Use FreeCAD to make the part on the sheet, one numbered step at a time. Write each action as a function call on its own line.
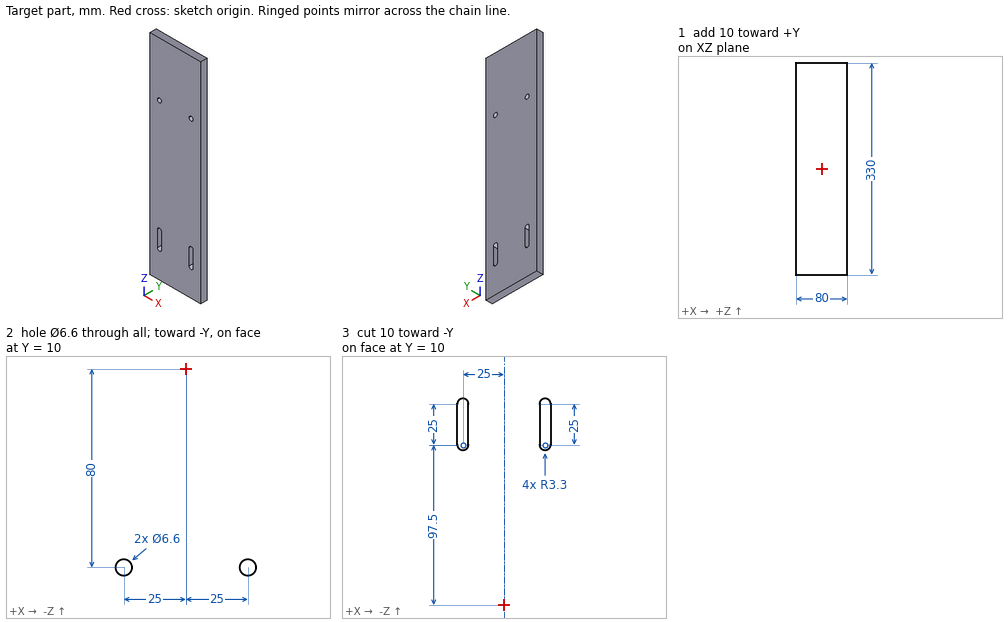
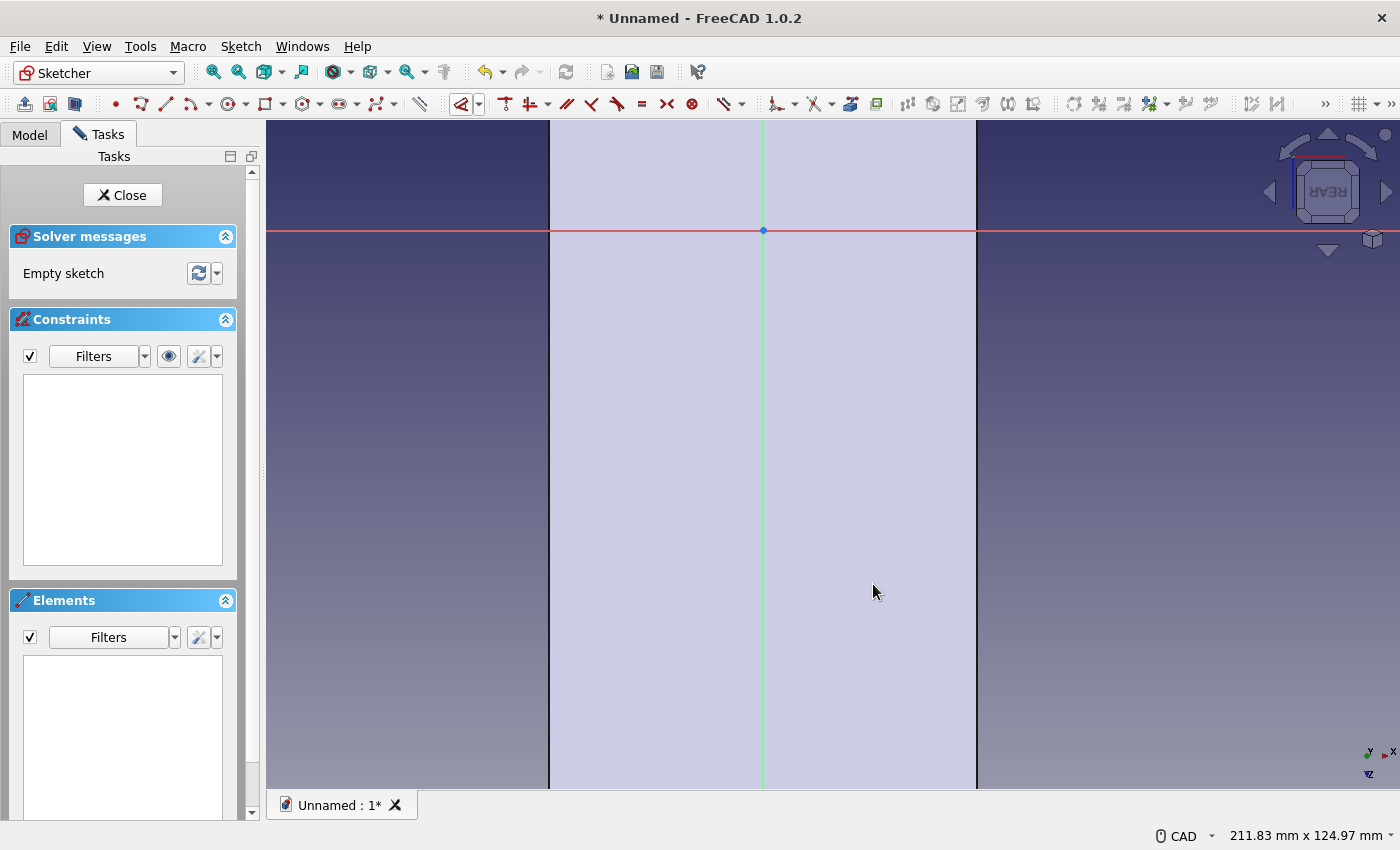
click(228, 104)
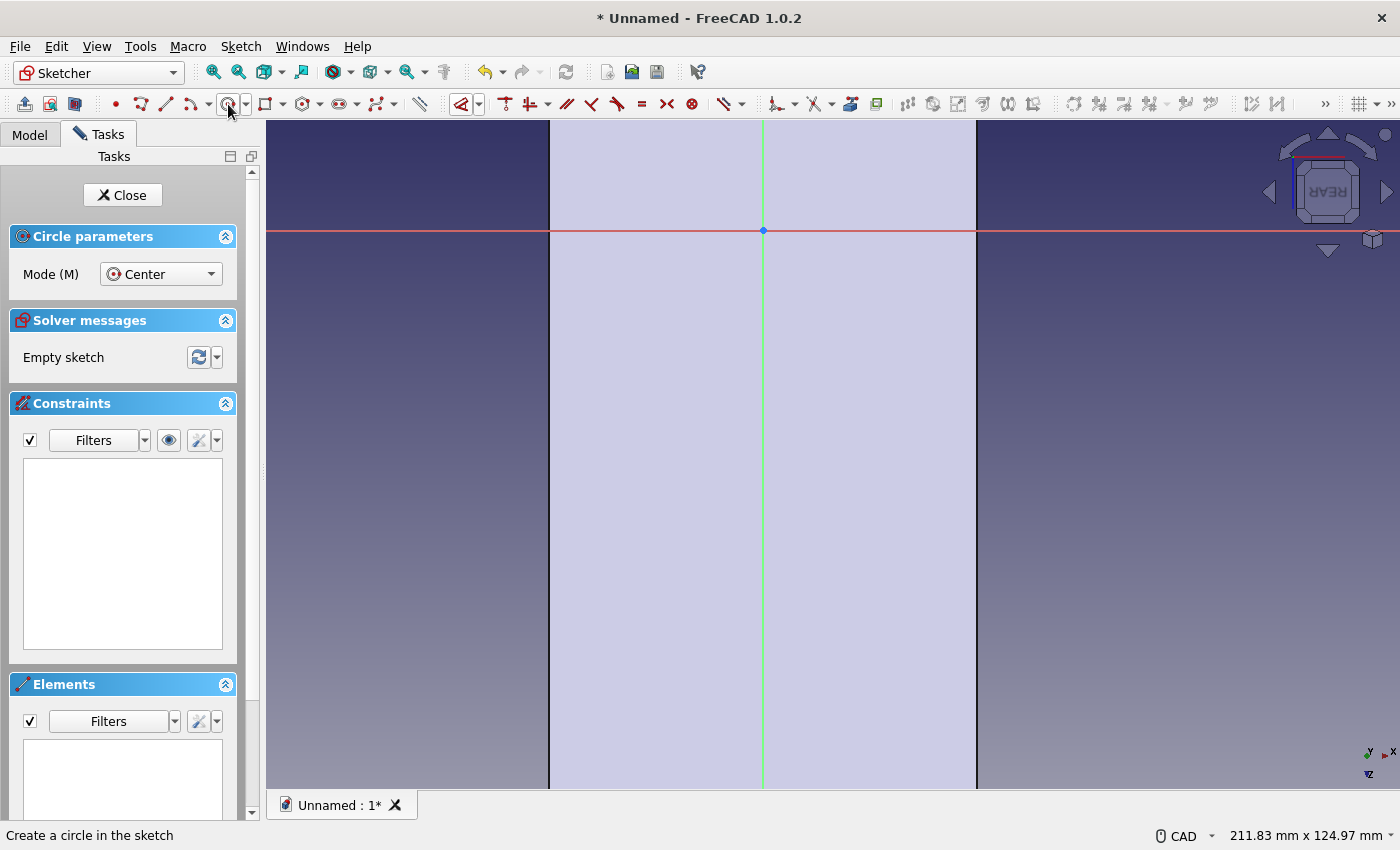
scroll(630, 659, up, 2)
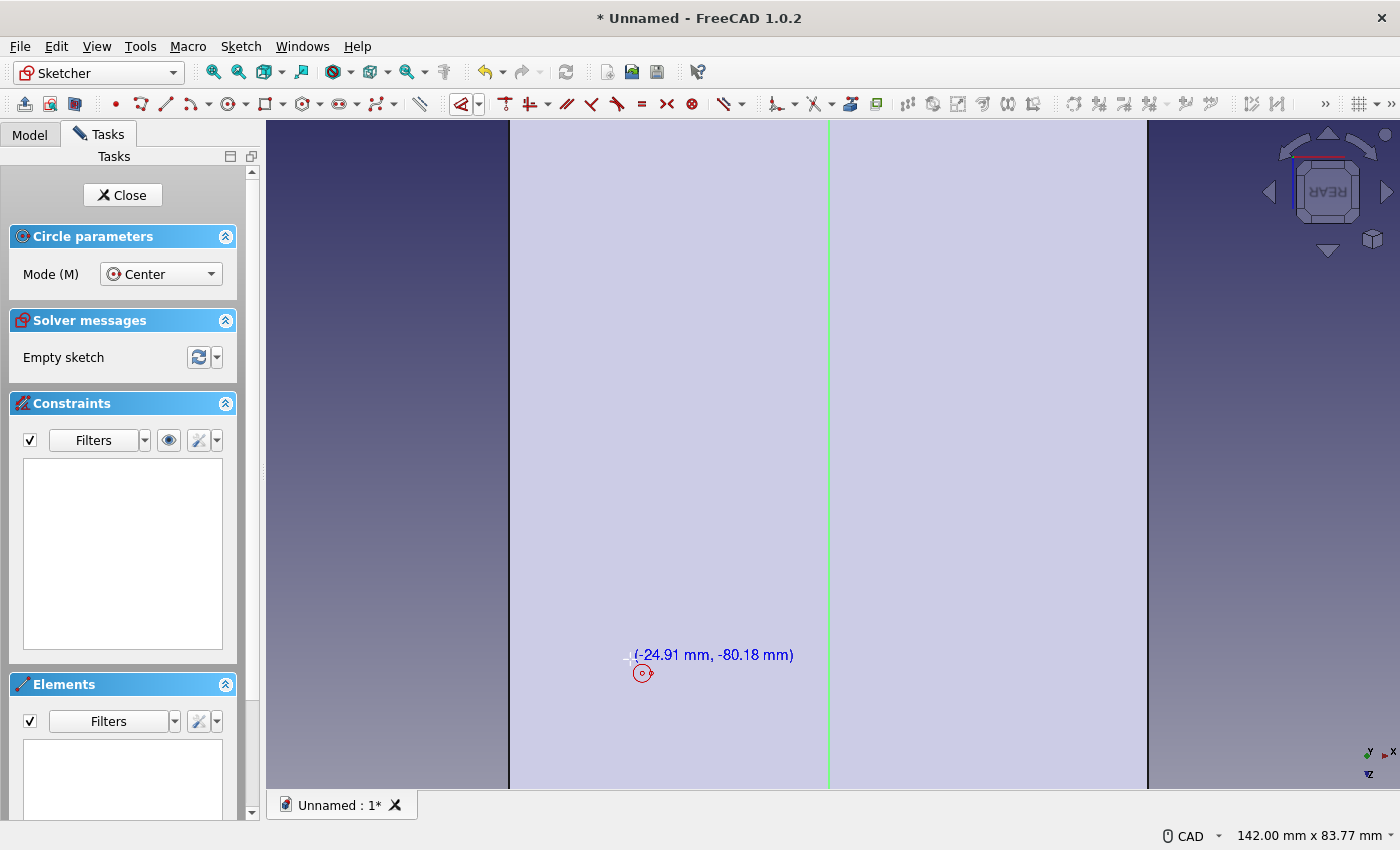
click(629, 659)
move(648, 640)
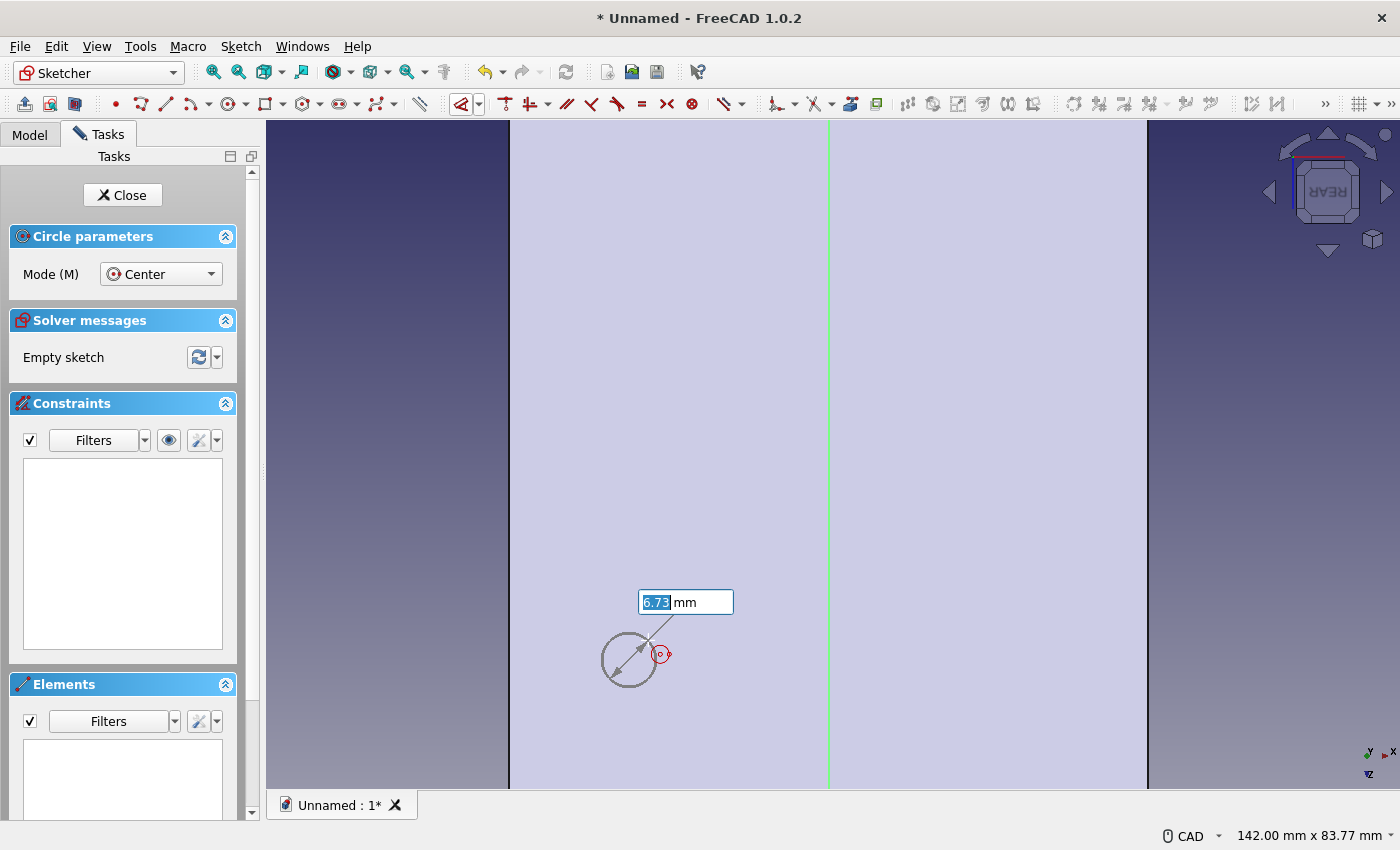
text(6.6)
key(Return)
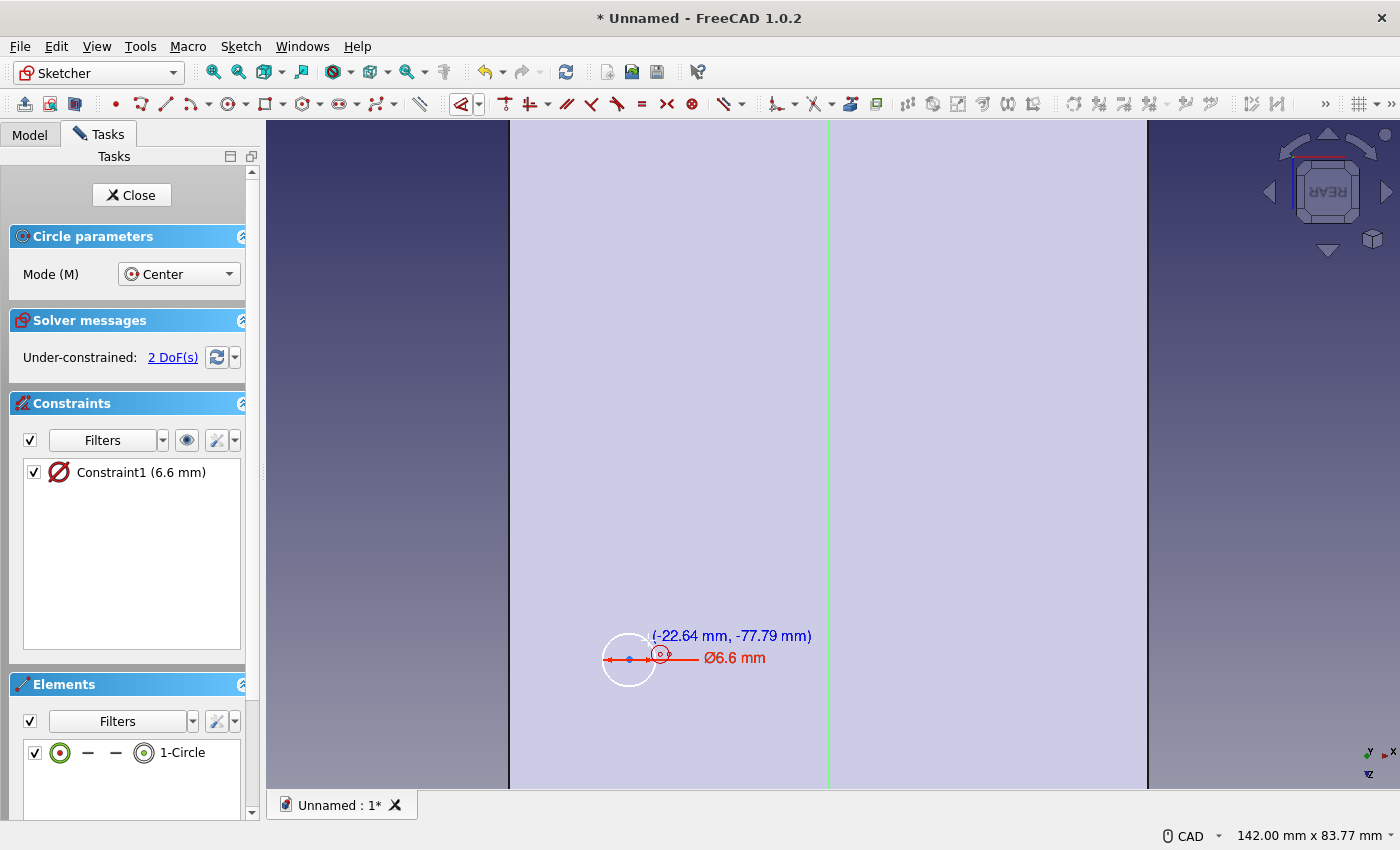
click(1028, 659)
move(1047, 640)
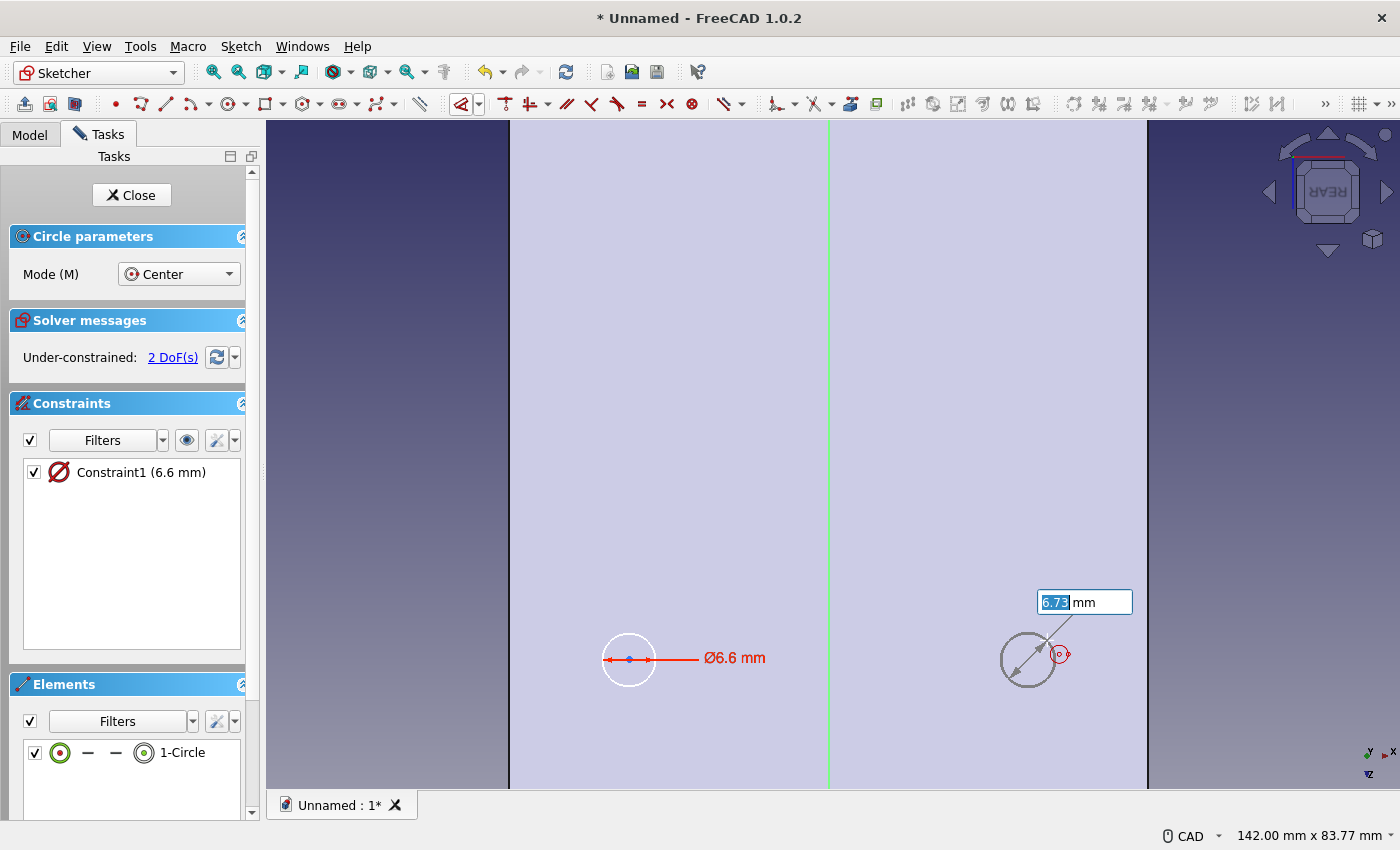
text(6.6)
key(Return)
key(Escape)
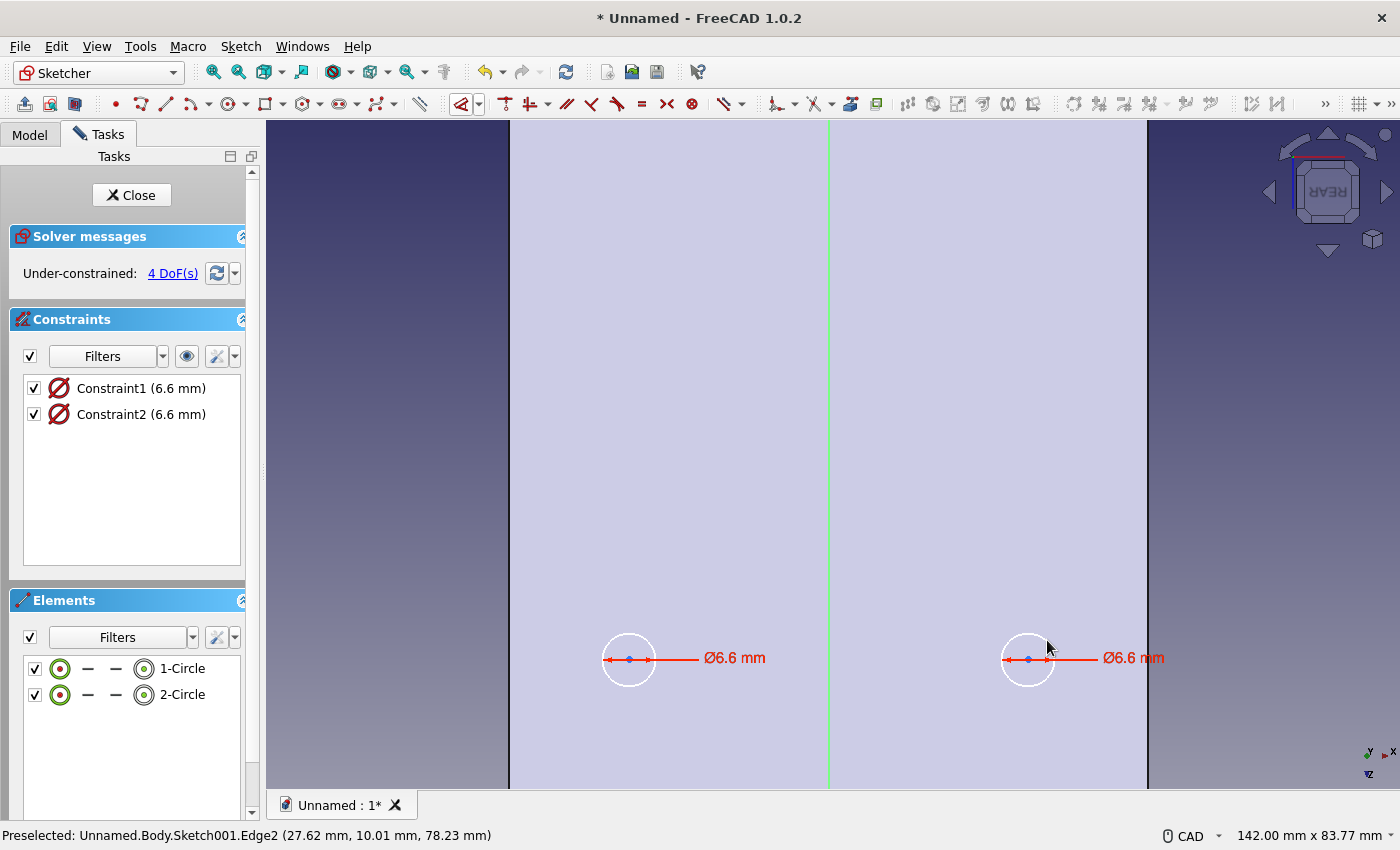
click(629, 660)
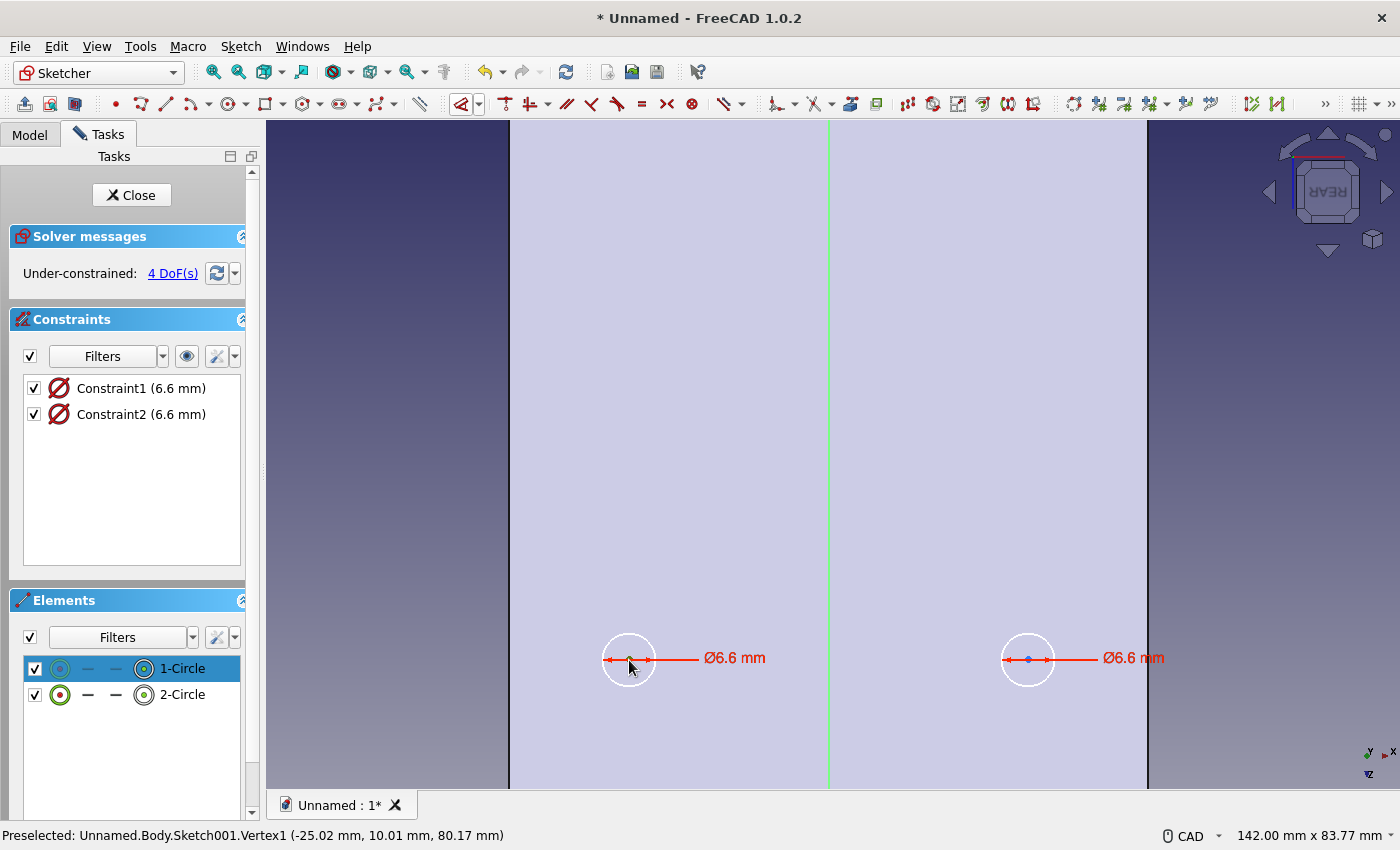
click(1028, 660)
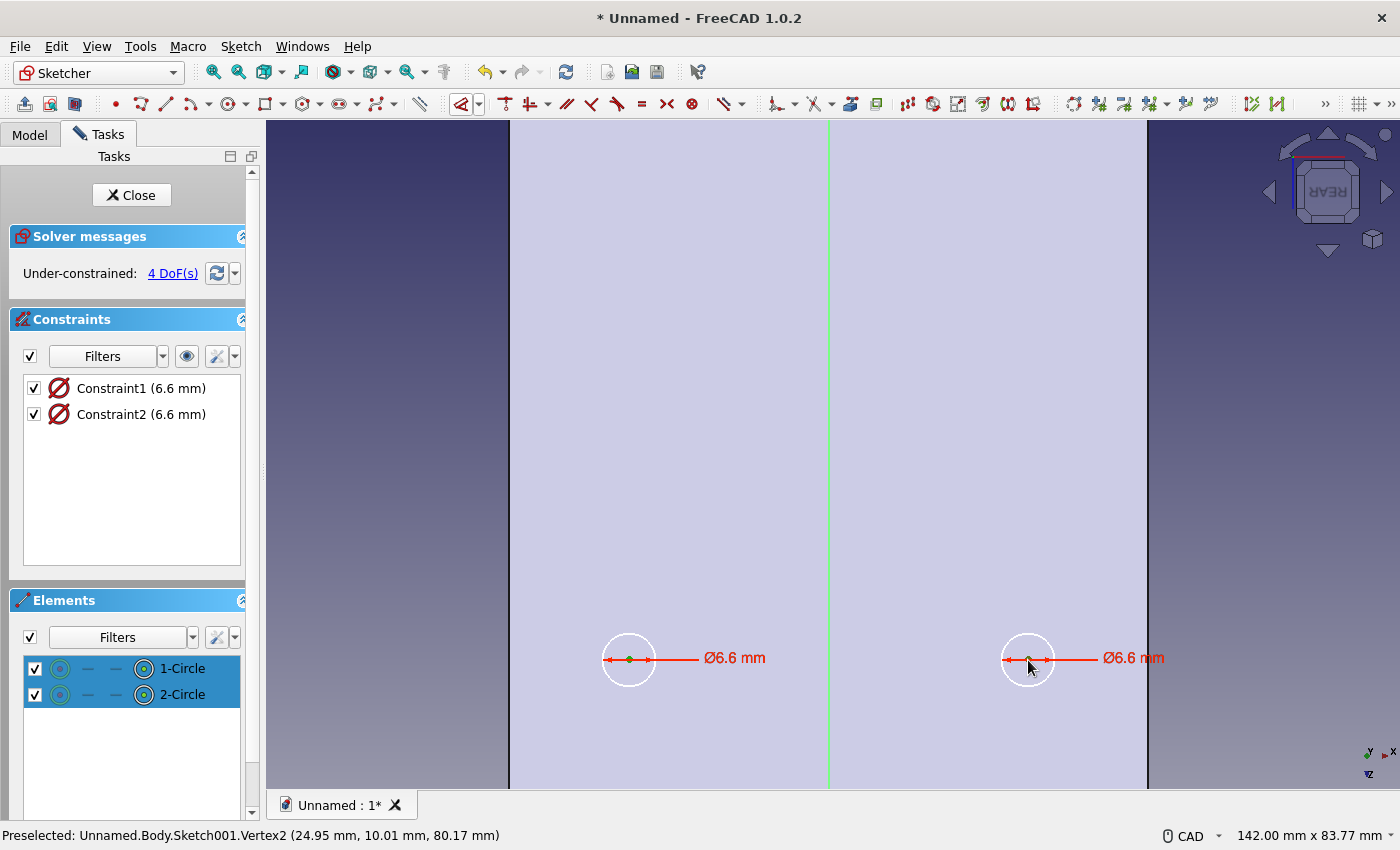
key(h)